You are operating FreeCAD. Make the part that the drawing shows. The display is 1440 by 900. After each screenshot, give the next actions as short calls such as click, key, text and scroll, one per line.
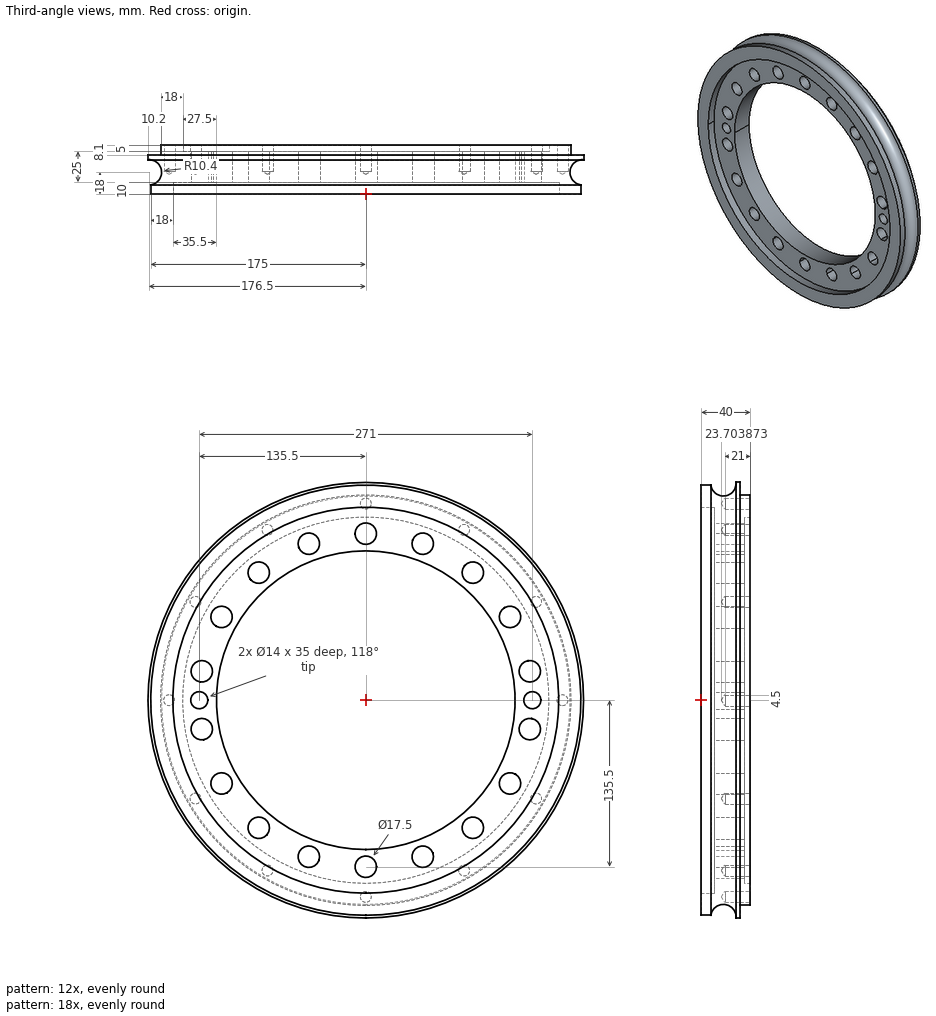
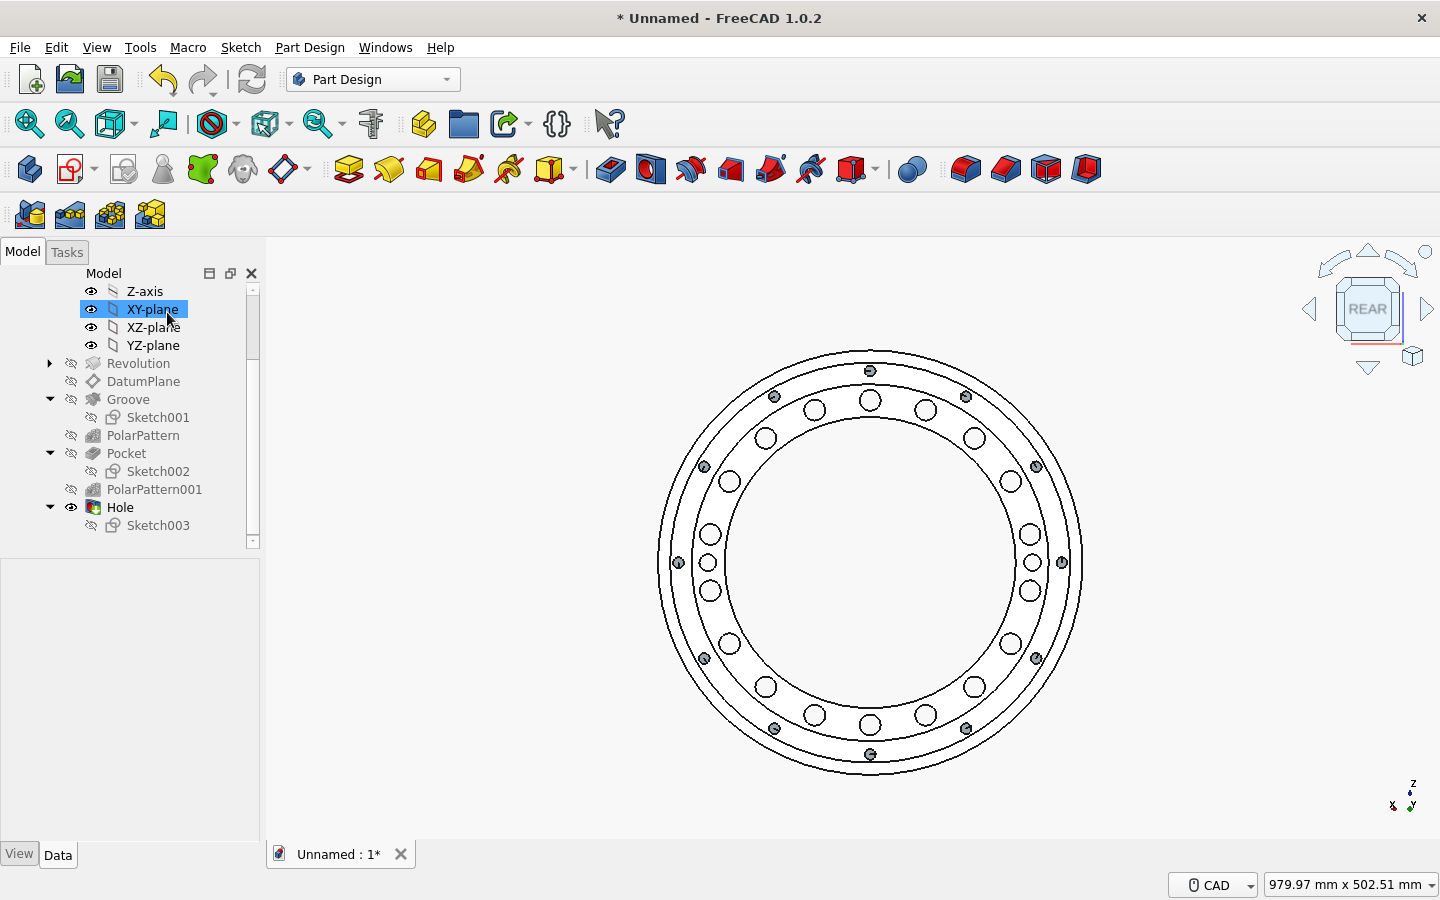
key(0)